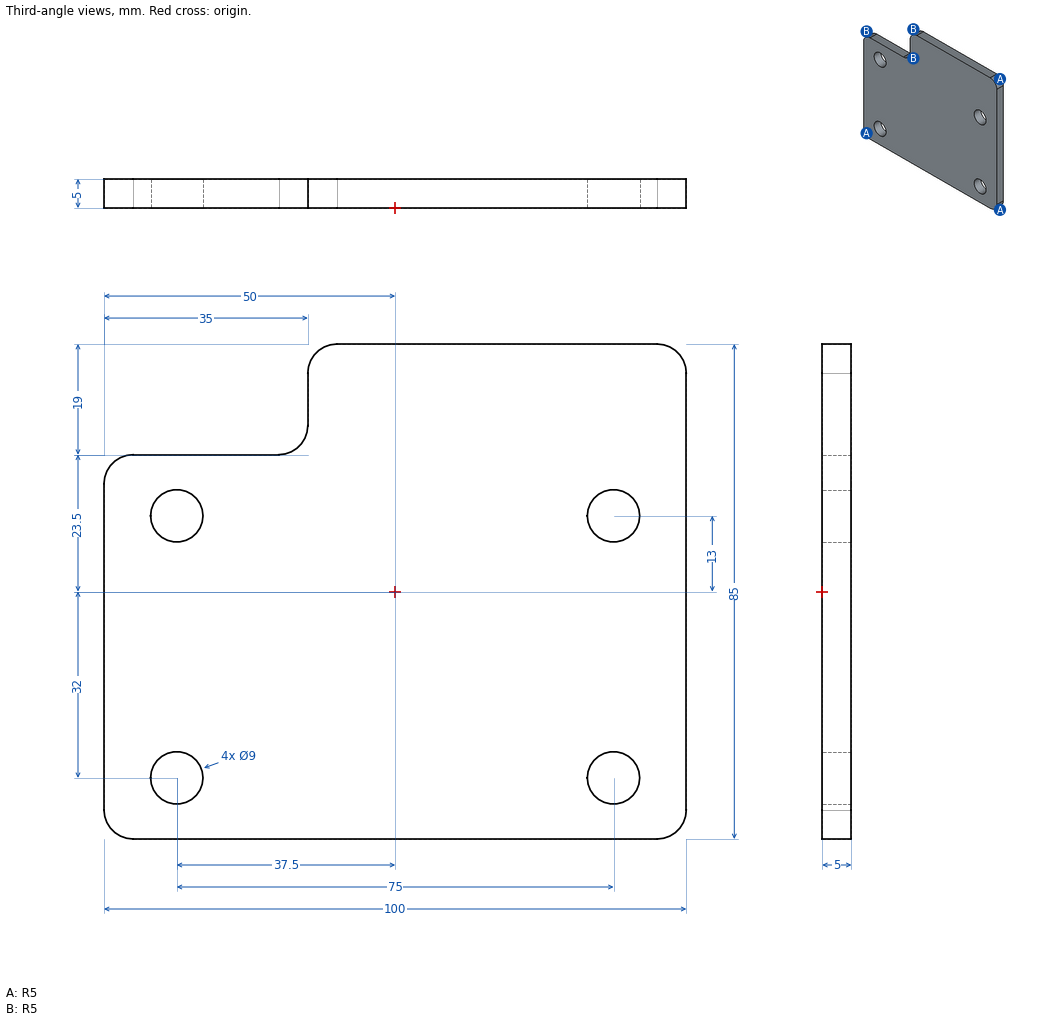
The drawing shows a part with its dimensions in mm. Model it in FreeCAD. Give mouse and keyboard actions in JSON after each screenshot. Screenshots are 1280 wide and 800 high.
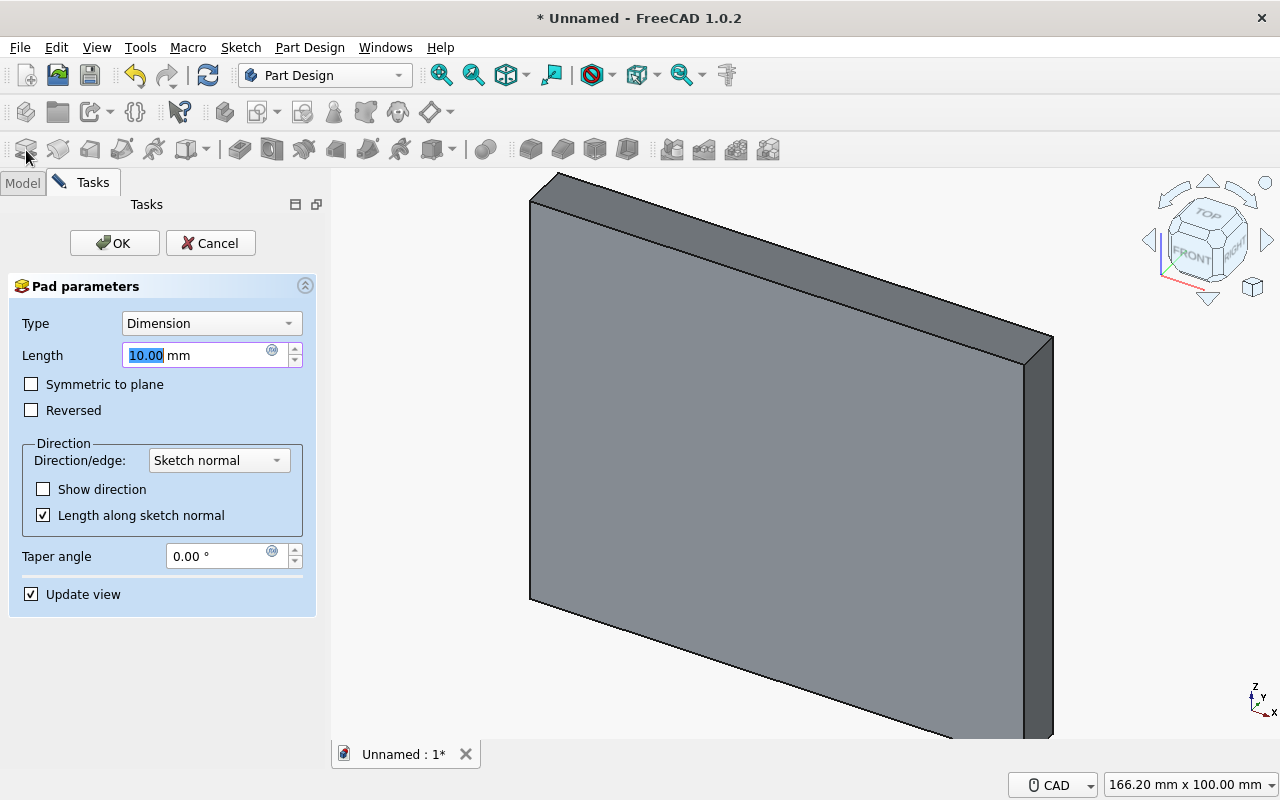
{"action": "type", "text": "5"}
{"action": "key", "text": "Tab"}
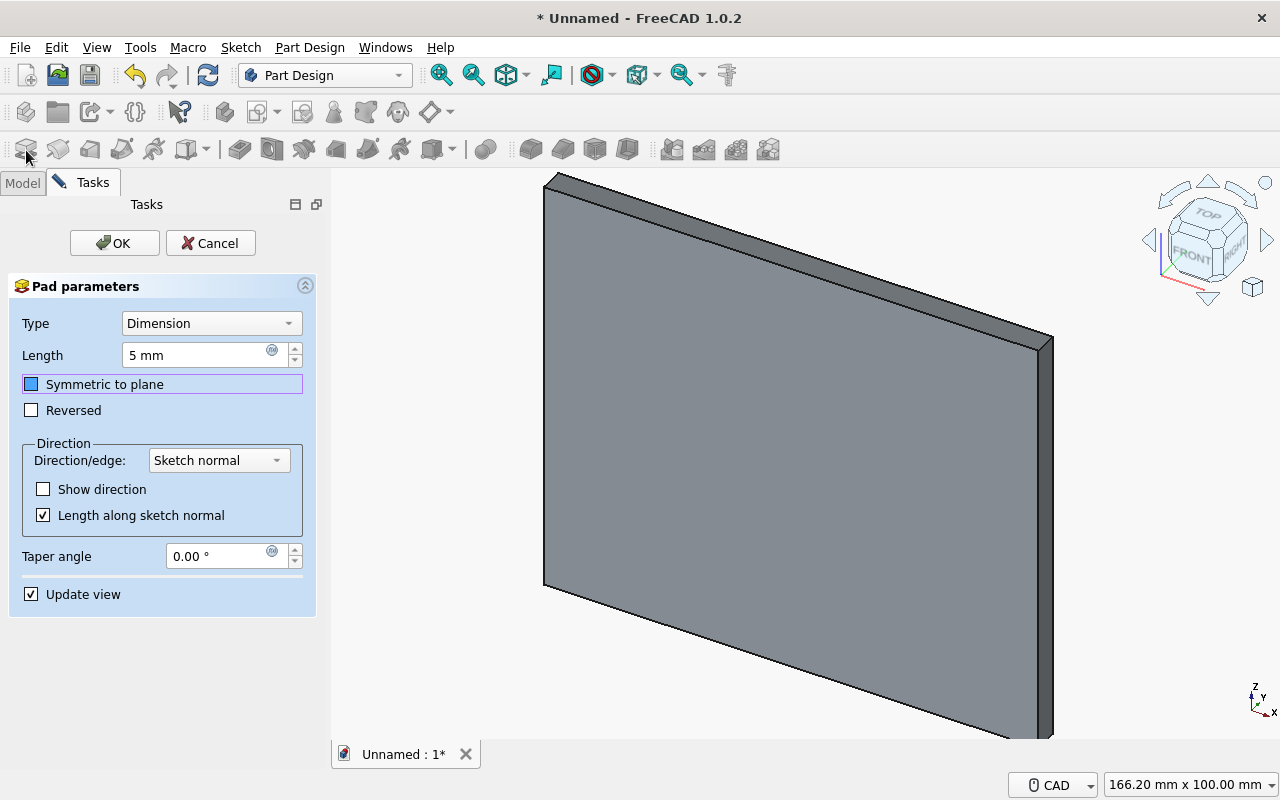
{"action": "left_click", "coordinate": [30, 410]}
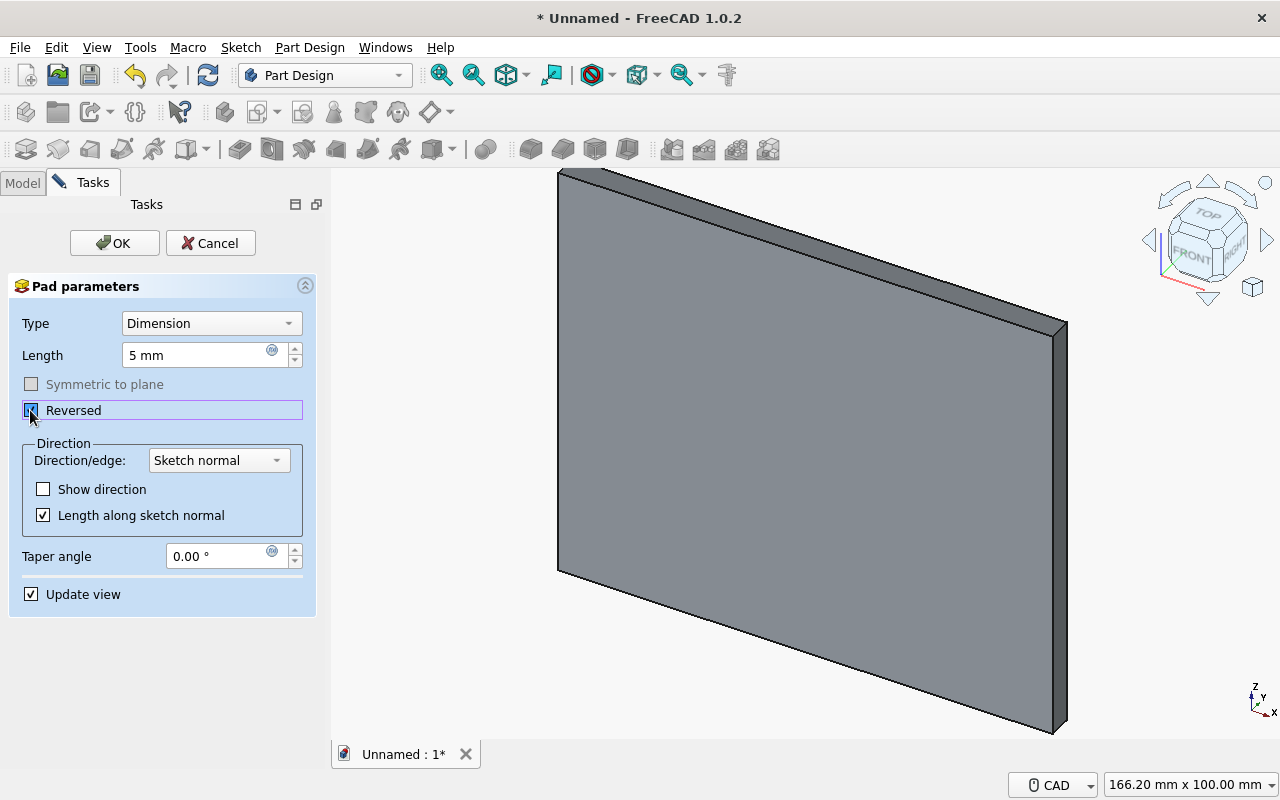
{"action": "left_click", "coordinate": [115, 243]}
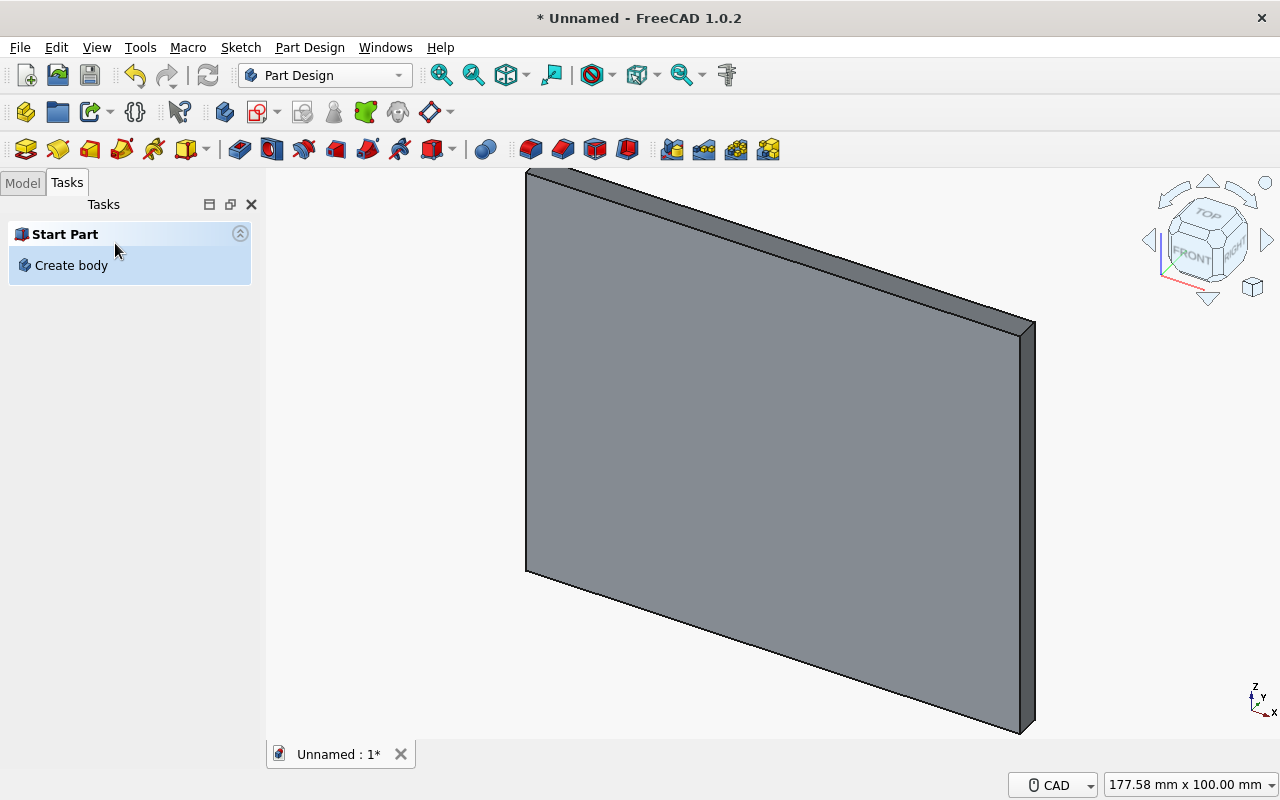
{"action": "left_click", "coordinate": [442, 76]}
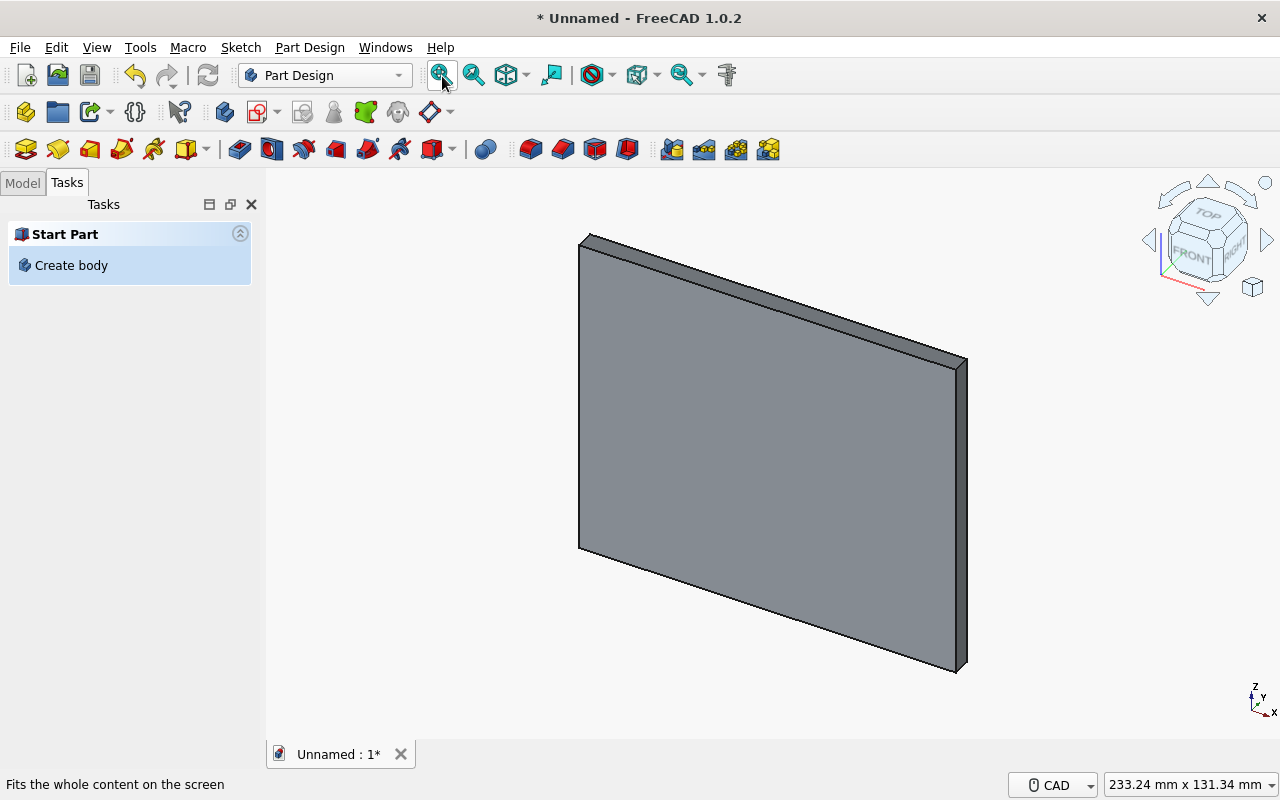
{"action": "key", "text": "4"}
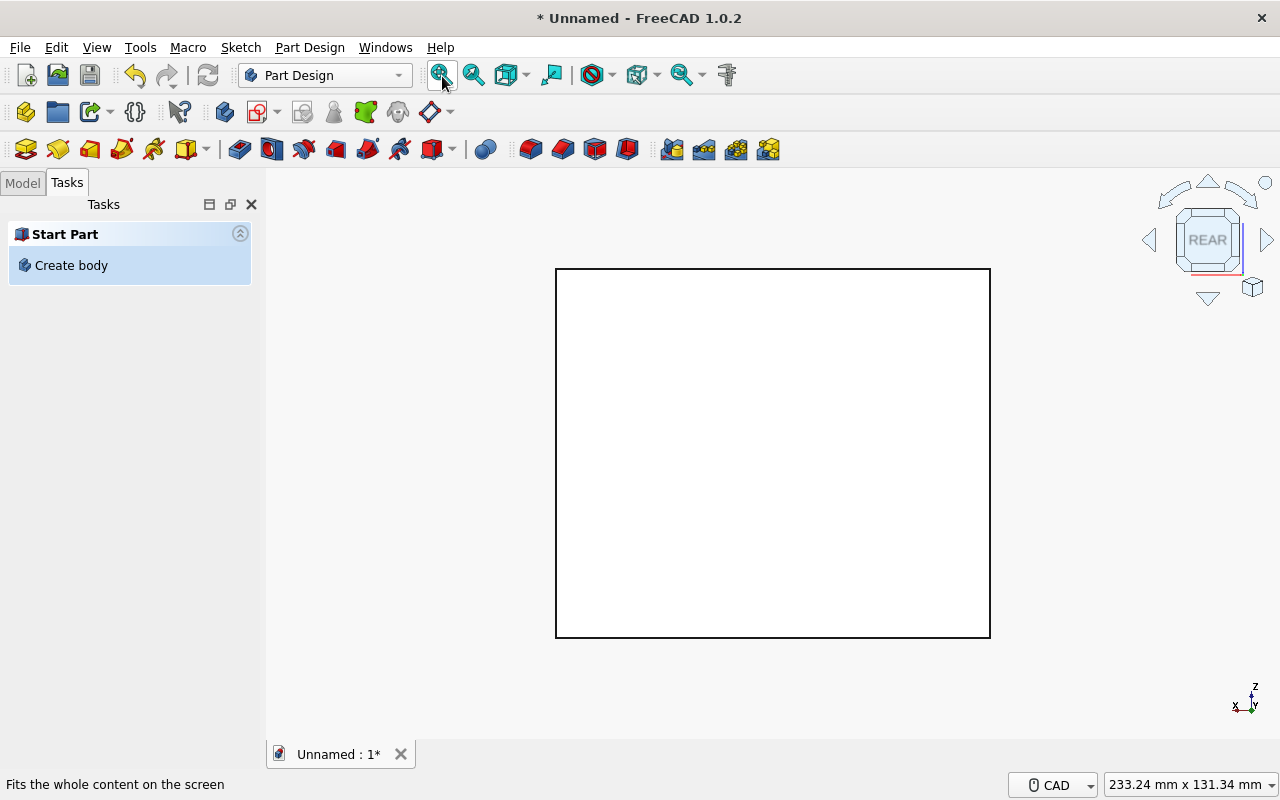
{"action": "left_click", "coordinate": [773, 453]}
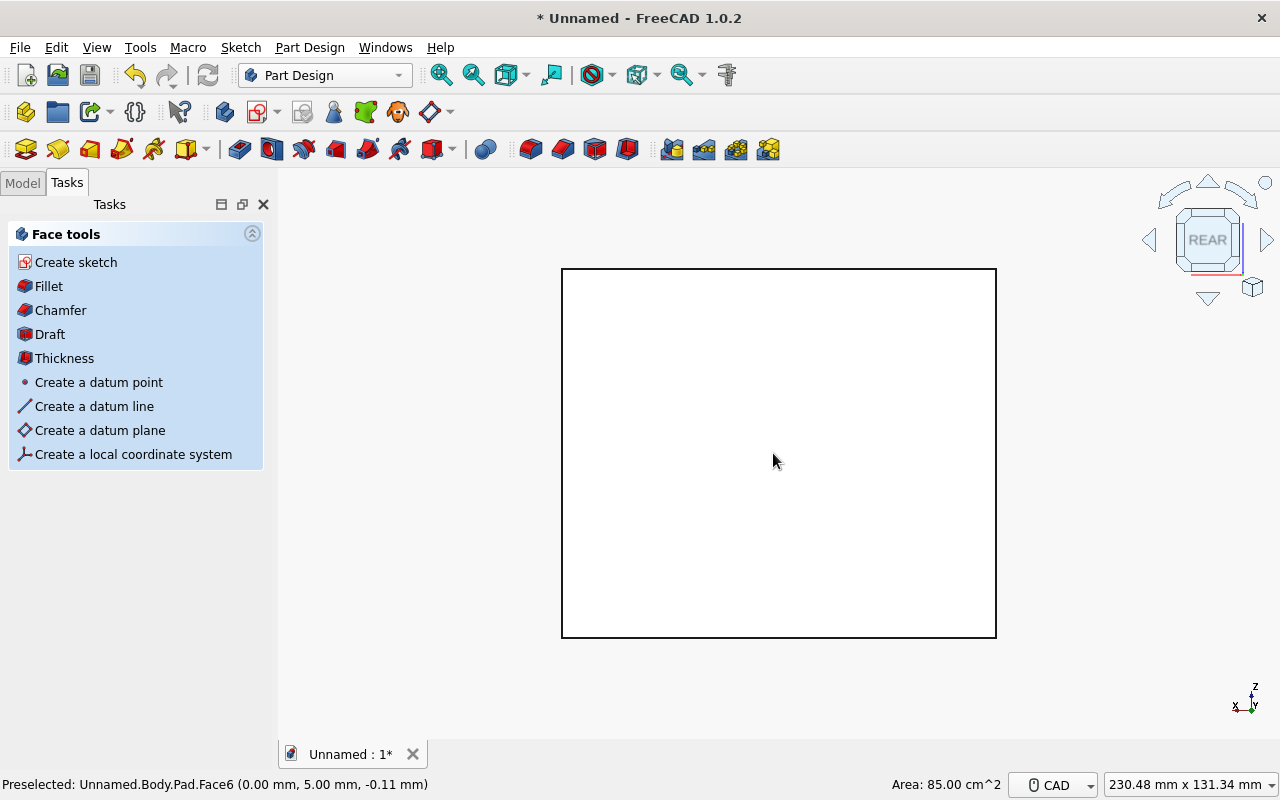
{"action": "left_click", "coordinate": [258, 112]}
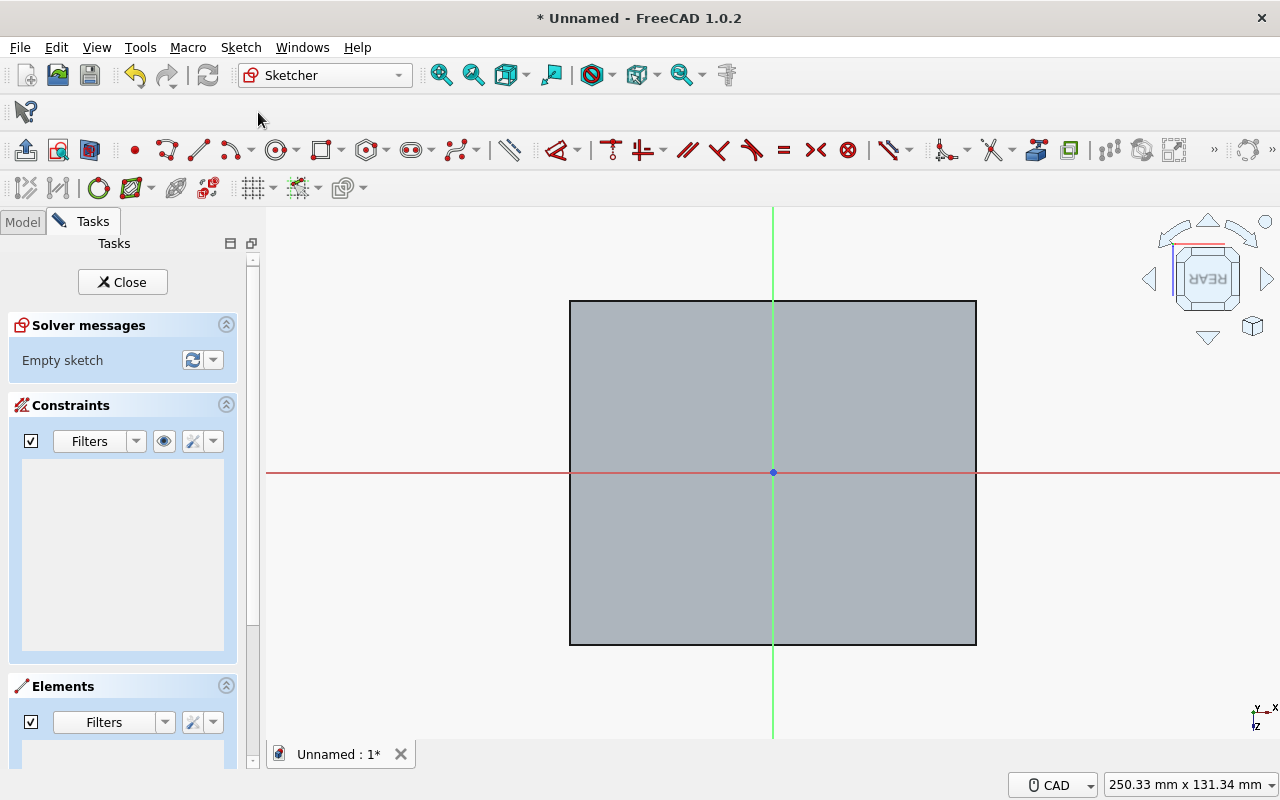
{"action": "scroll", "coordinate": [912, 356], "scroll_direction": "up", "scroll_amount": 2}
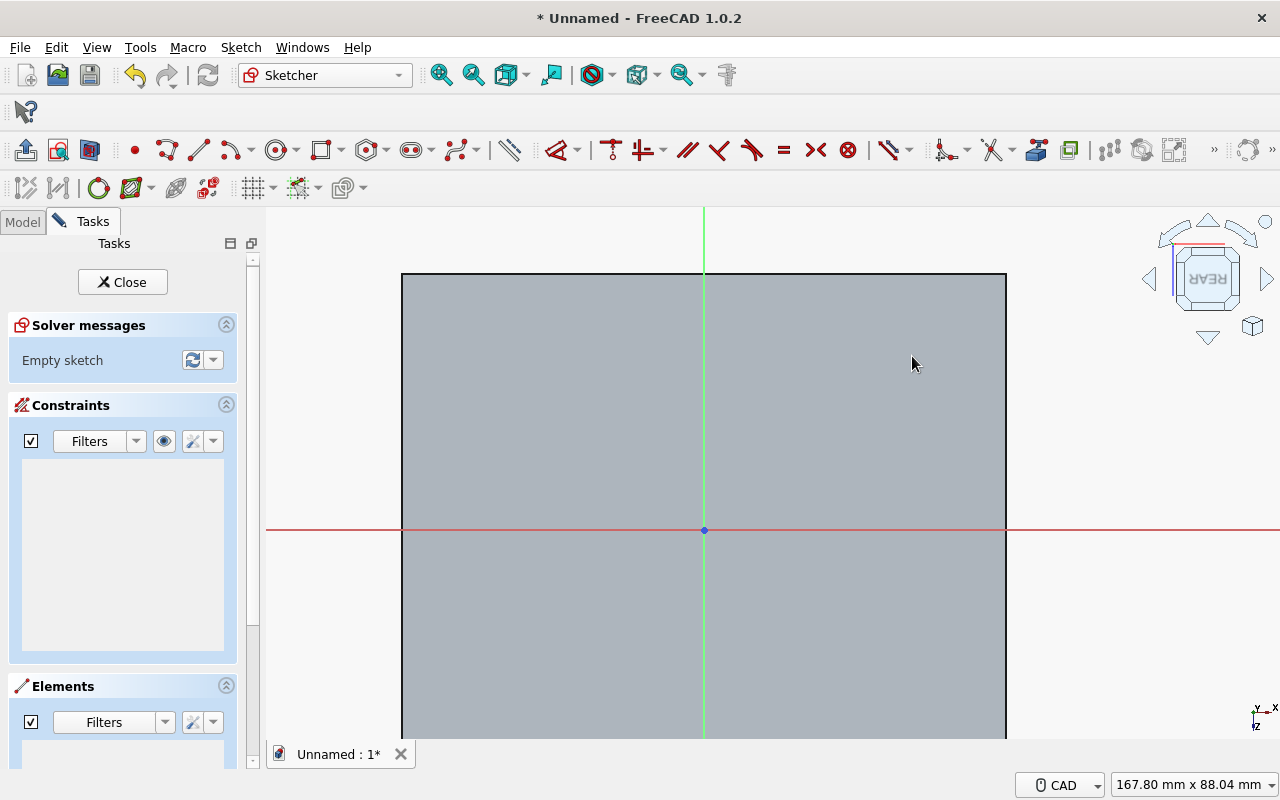
{"action": "left_click", "coordinate": [276, 150]}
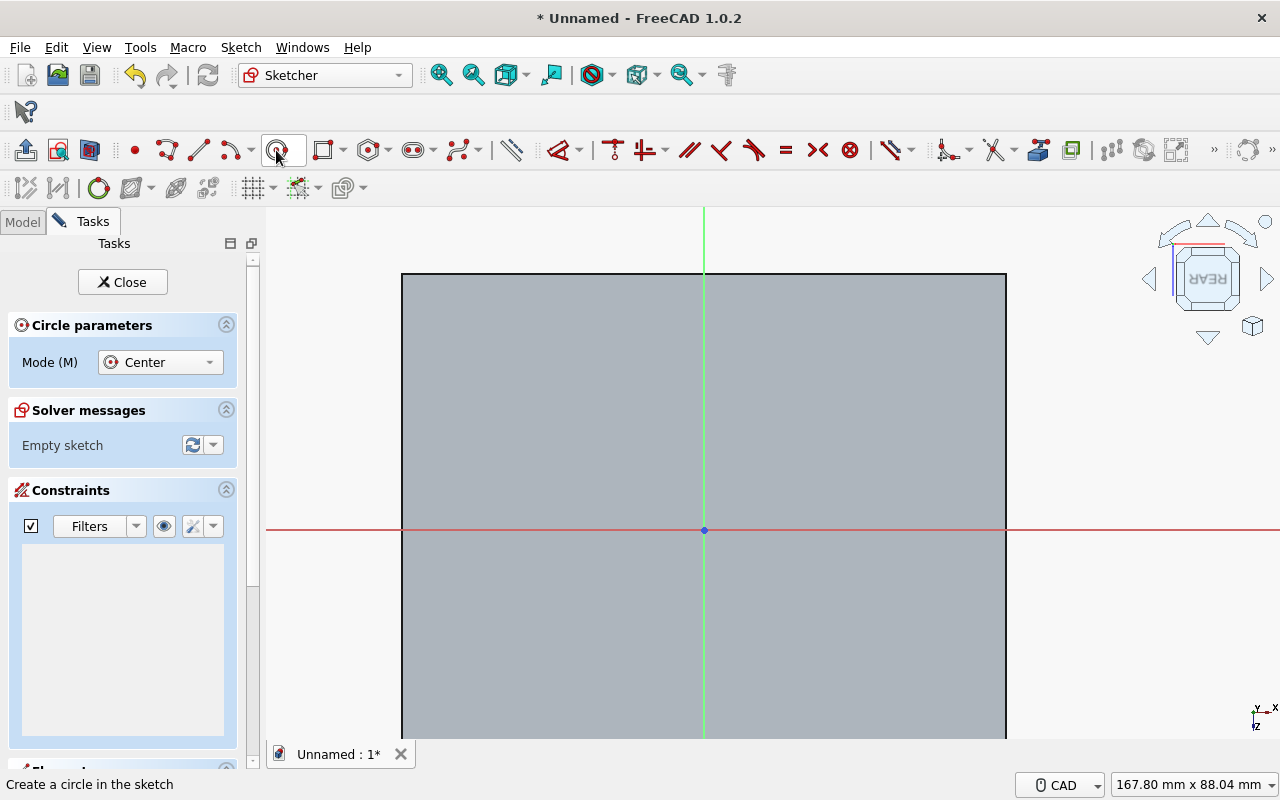
{"action": "left_click", "coordinate": [478, 337]}
{"action": "mouse_move", "coordinate": [497, 318]}